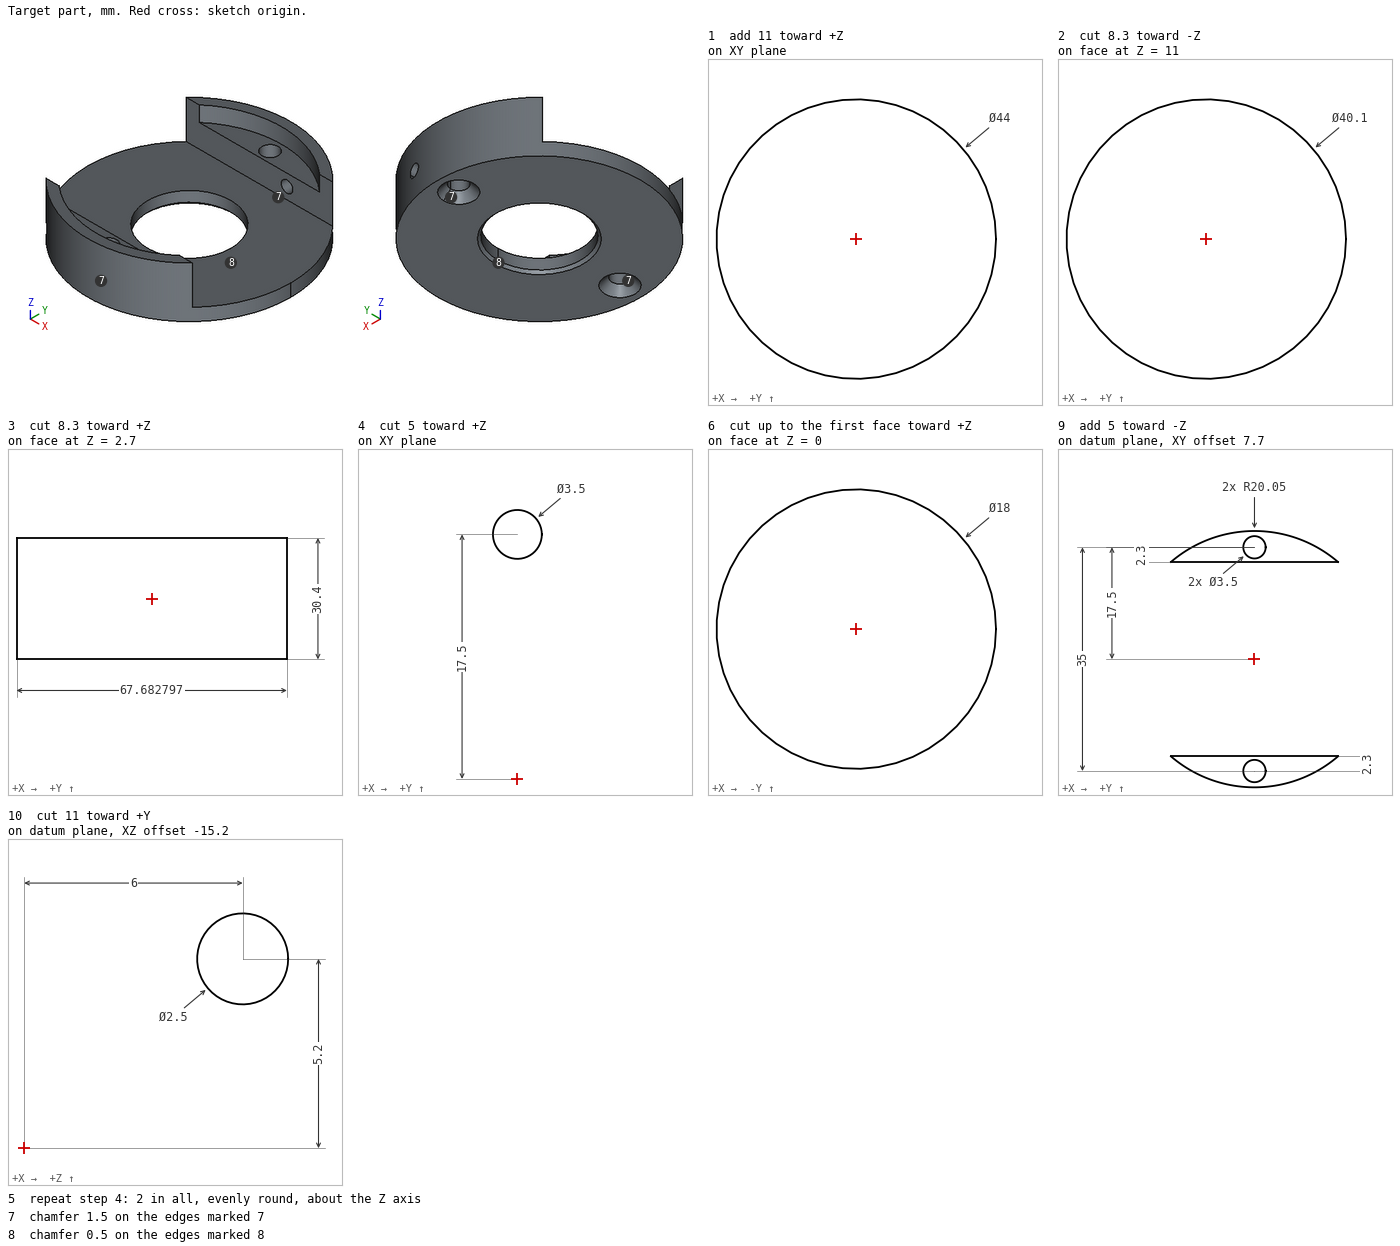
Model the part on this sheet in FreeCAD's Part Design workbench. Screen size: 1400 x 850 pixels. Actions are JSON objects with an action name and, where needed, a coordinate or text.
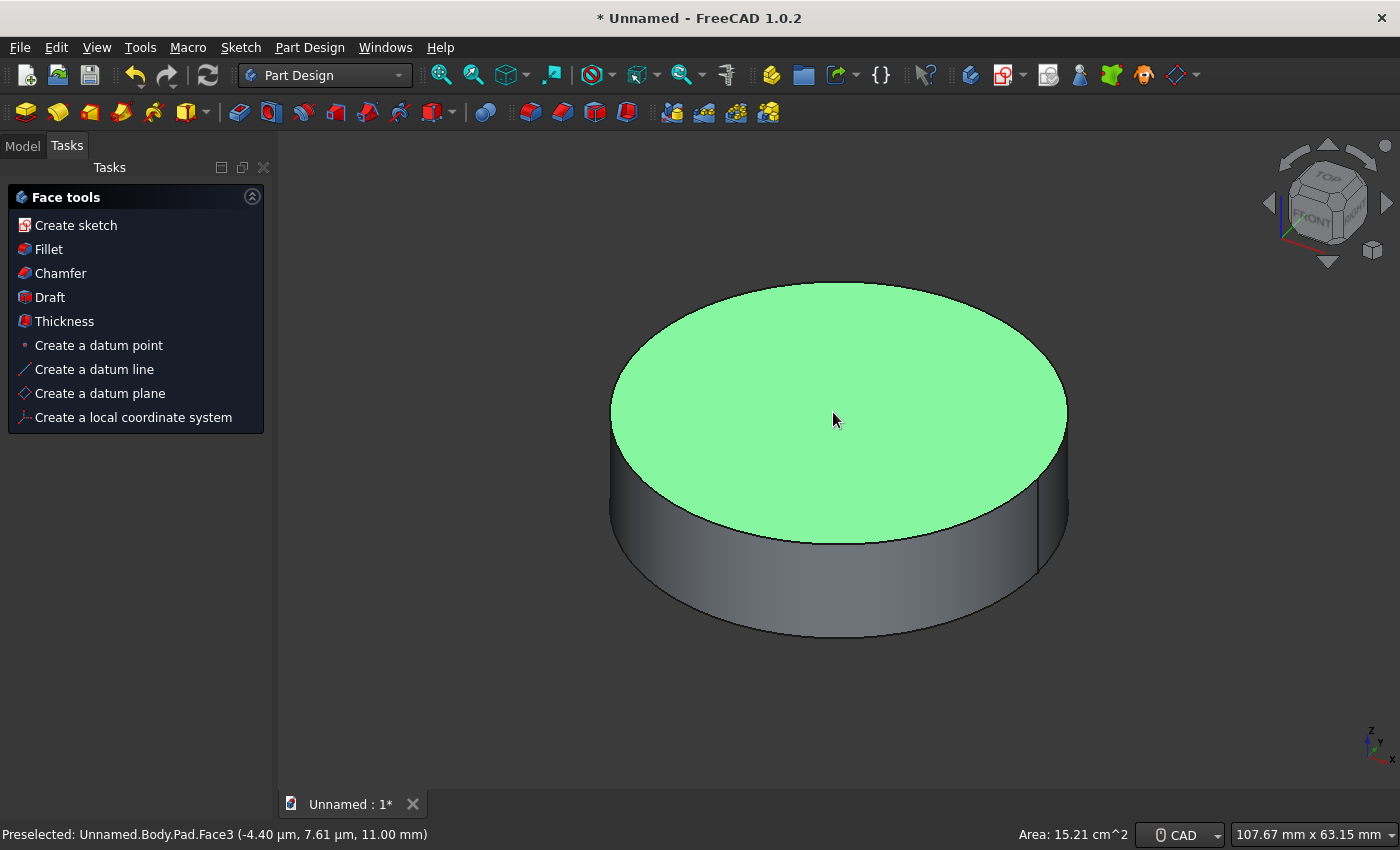
{"action": "left_click", "coordinate": [1004, 76]}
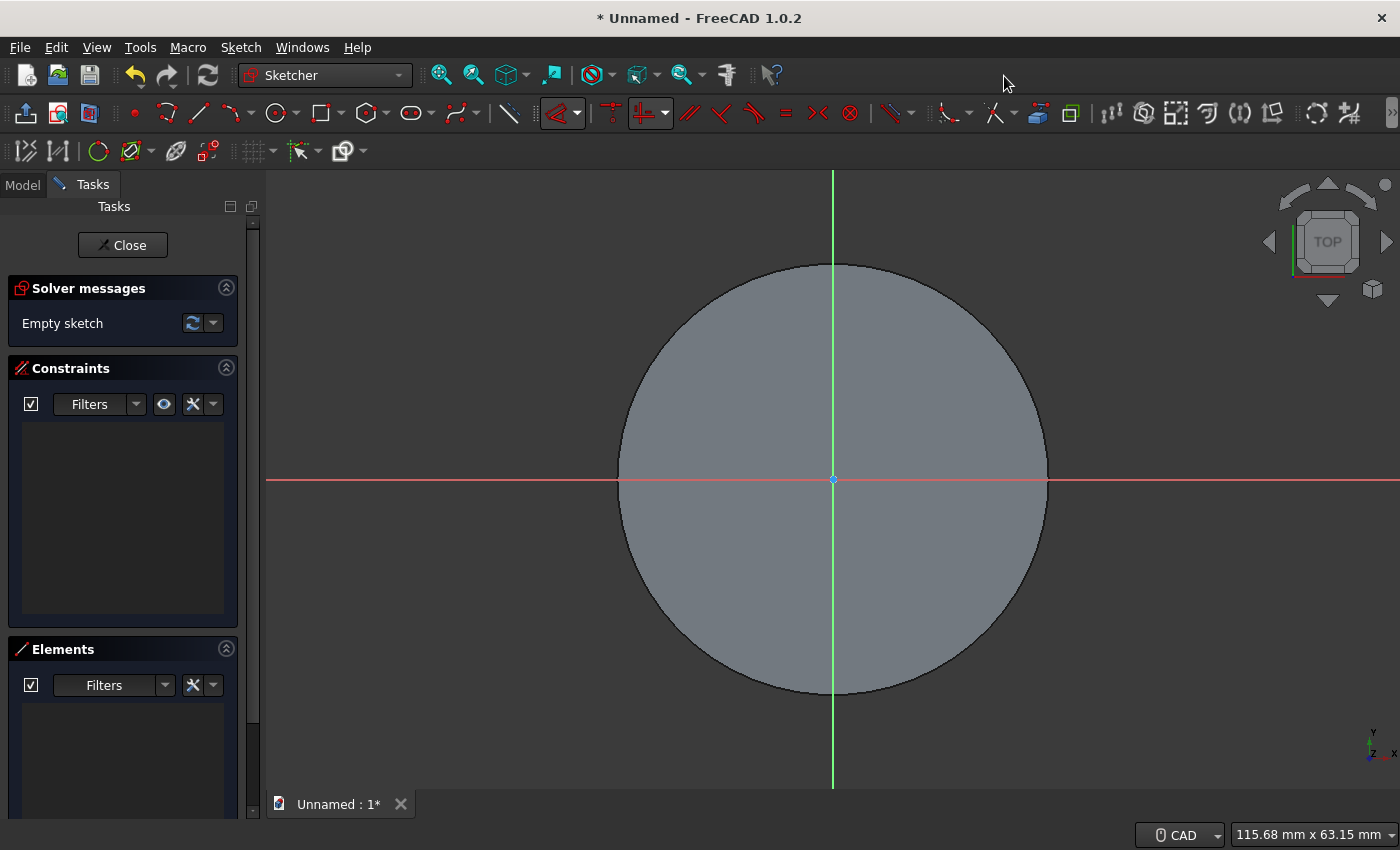
{"action": "key", "text": "g c"}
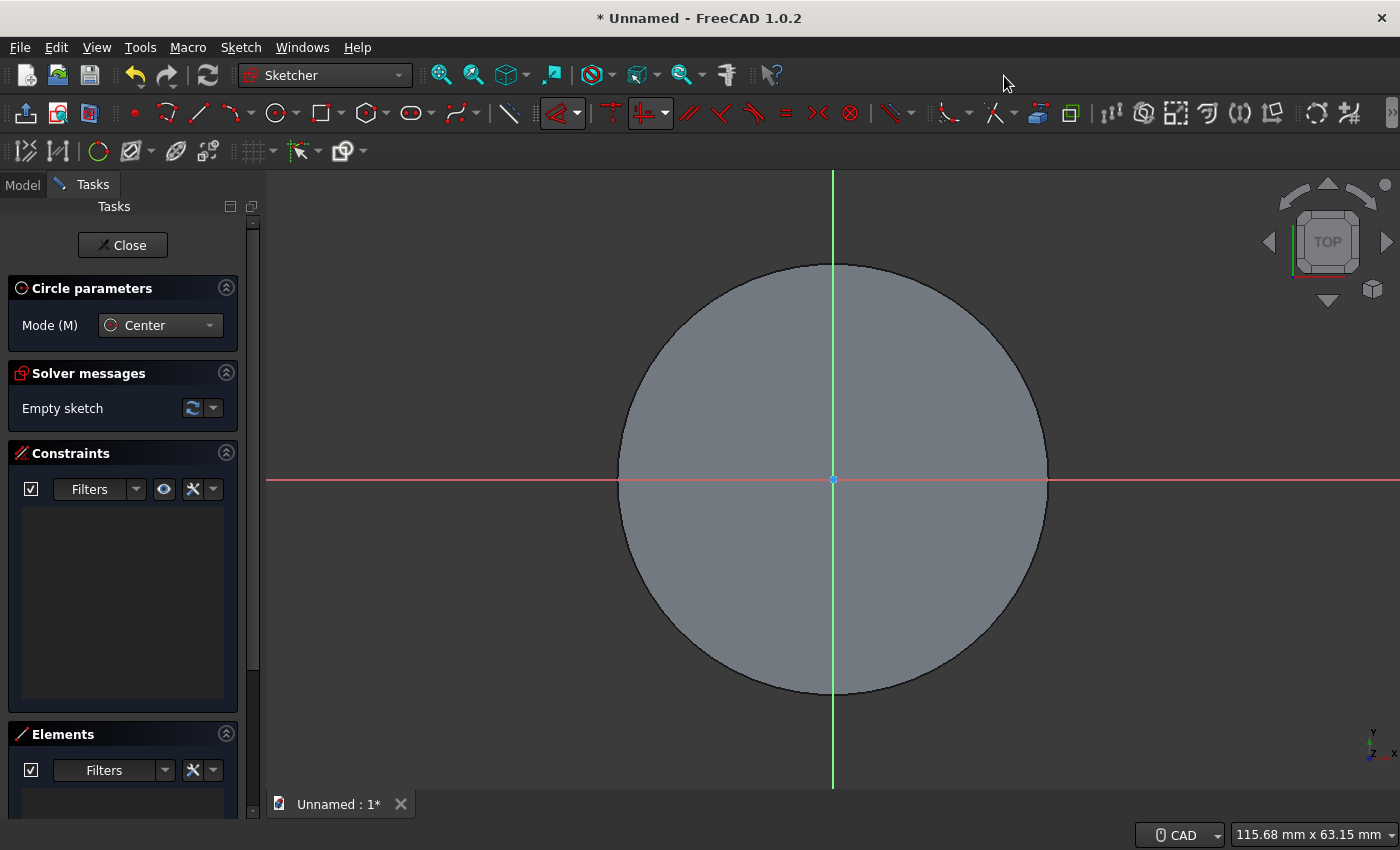
{"action": "left_click", "coordinate": [833, 480]}
{"action": "left_click", "coordinate": [972, 341]}
{"action": "key", "text": "Escape"}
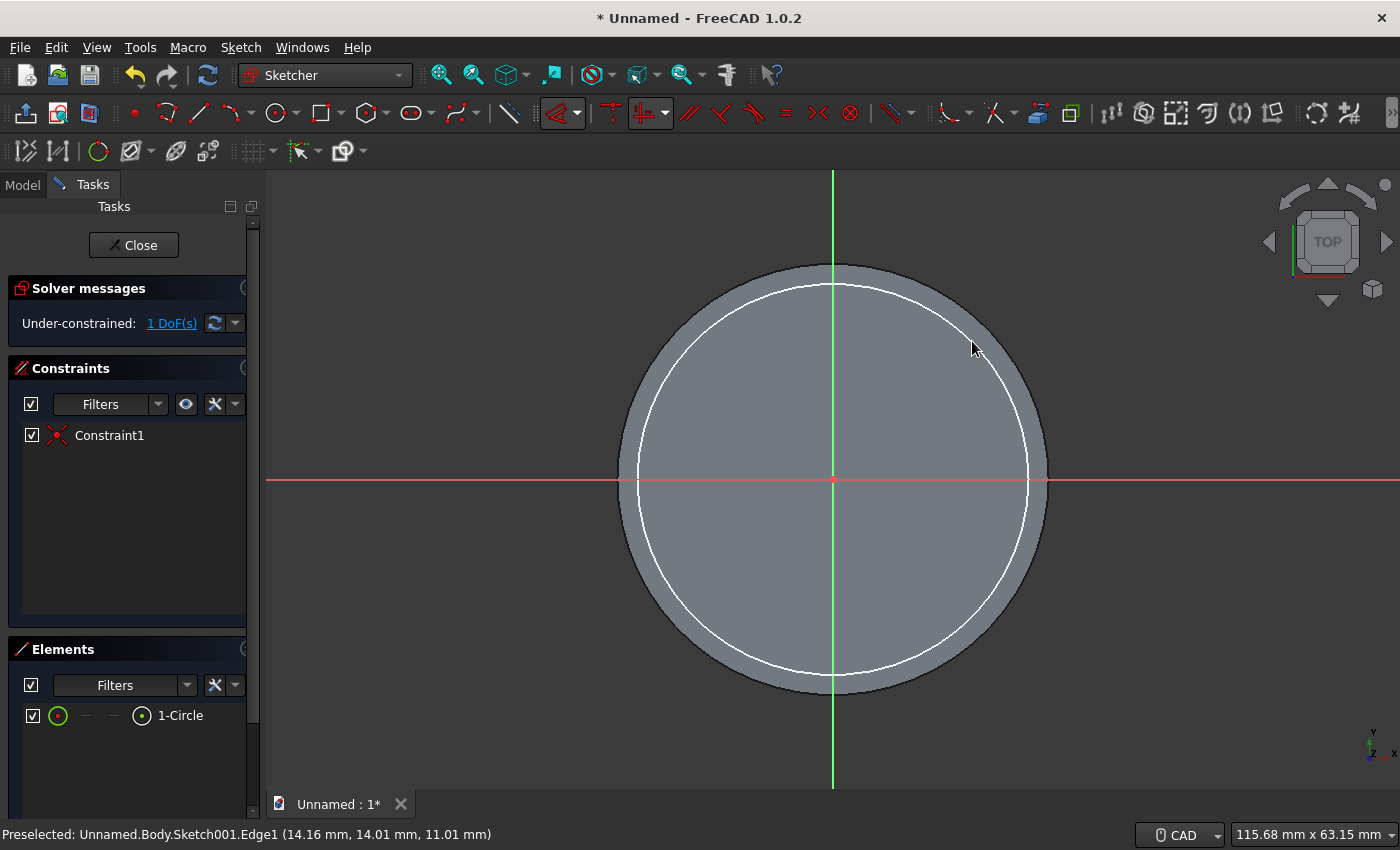
{"action": "left_click", "coordinate": [556, 114]}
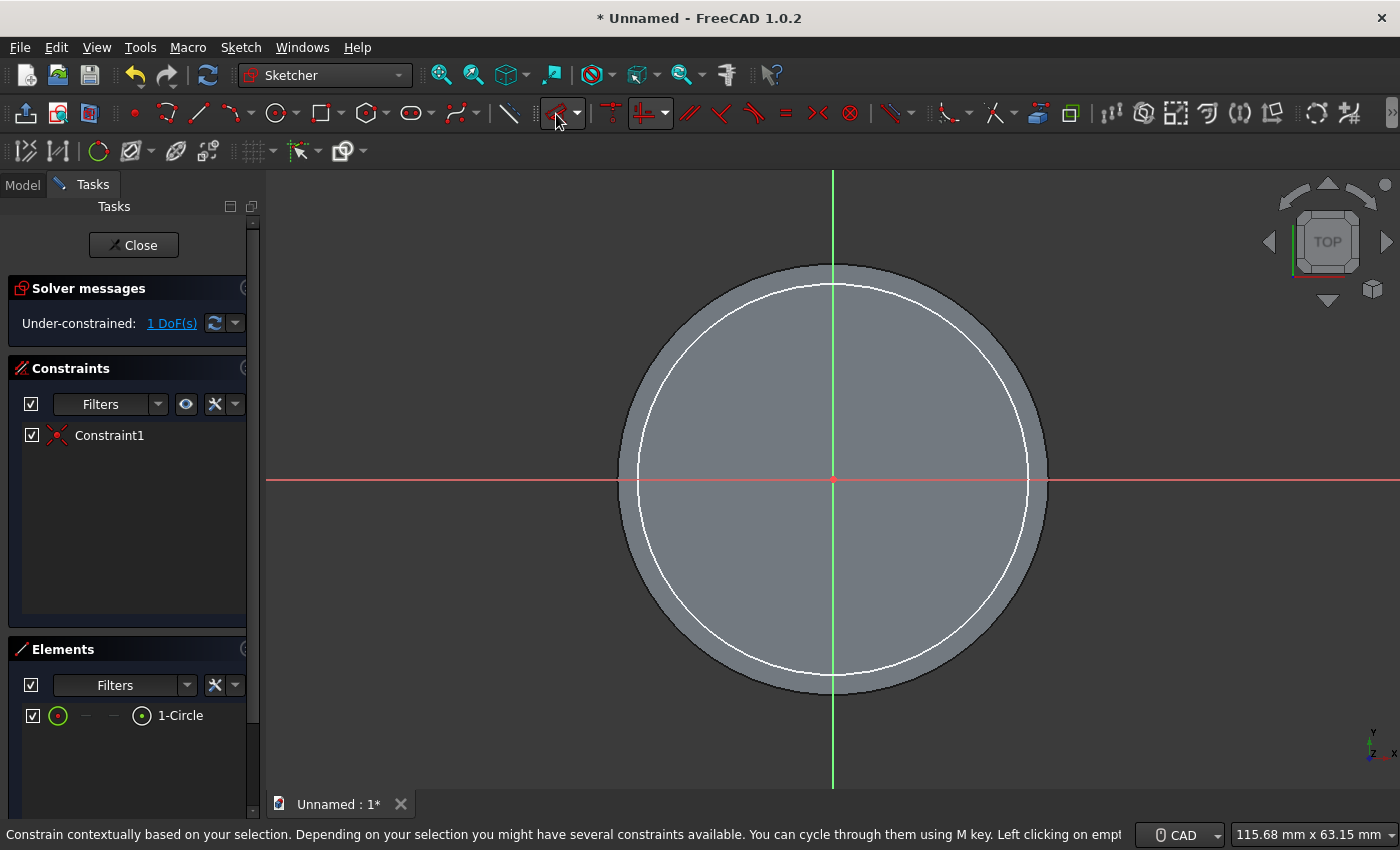
{"action": "left_click", "coordinate": [971, 341]}
{"action": "left_click", "coordinate": [994, 318]}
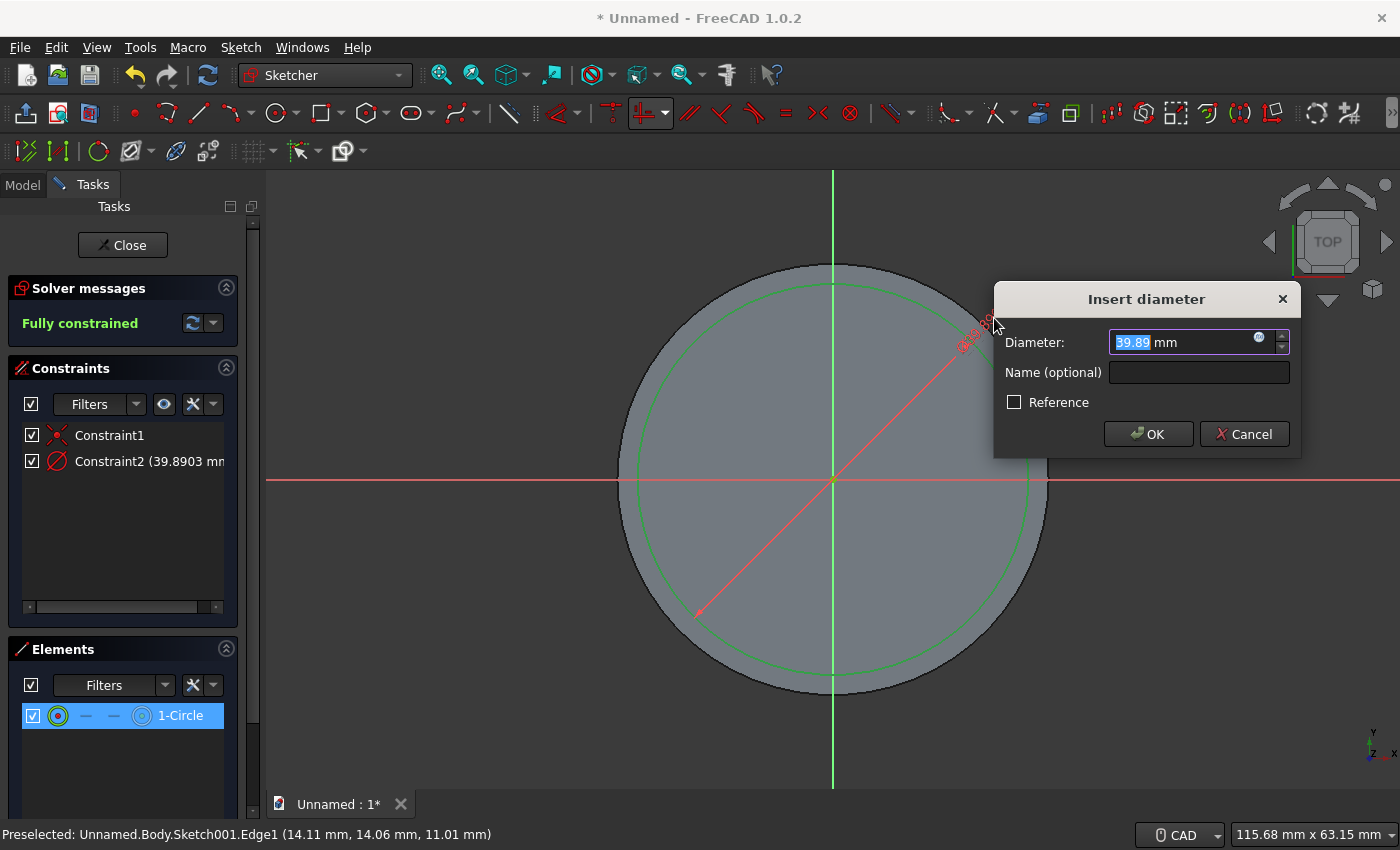
{"action": "type", "text": "40.1"}
{"action": "key", "text": "Return"}
{"action": "key", "text": "Escape"}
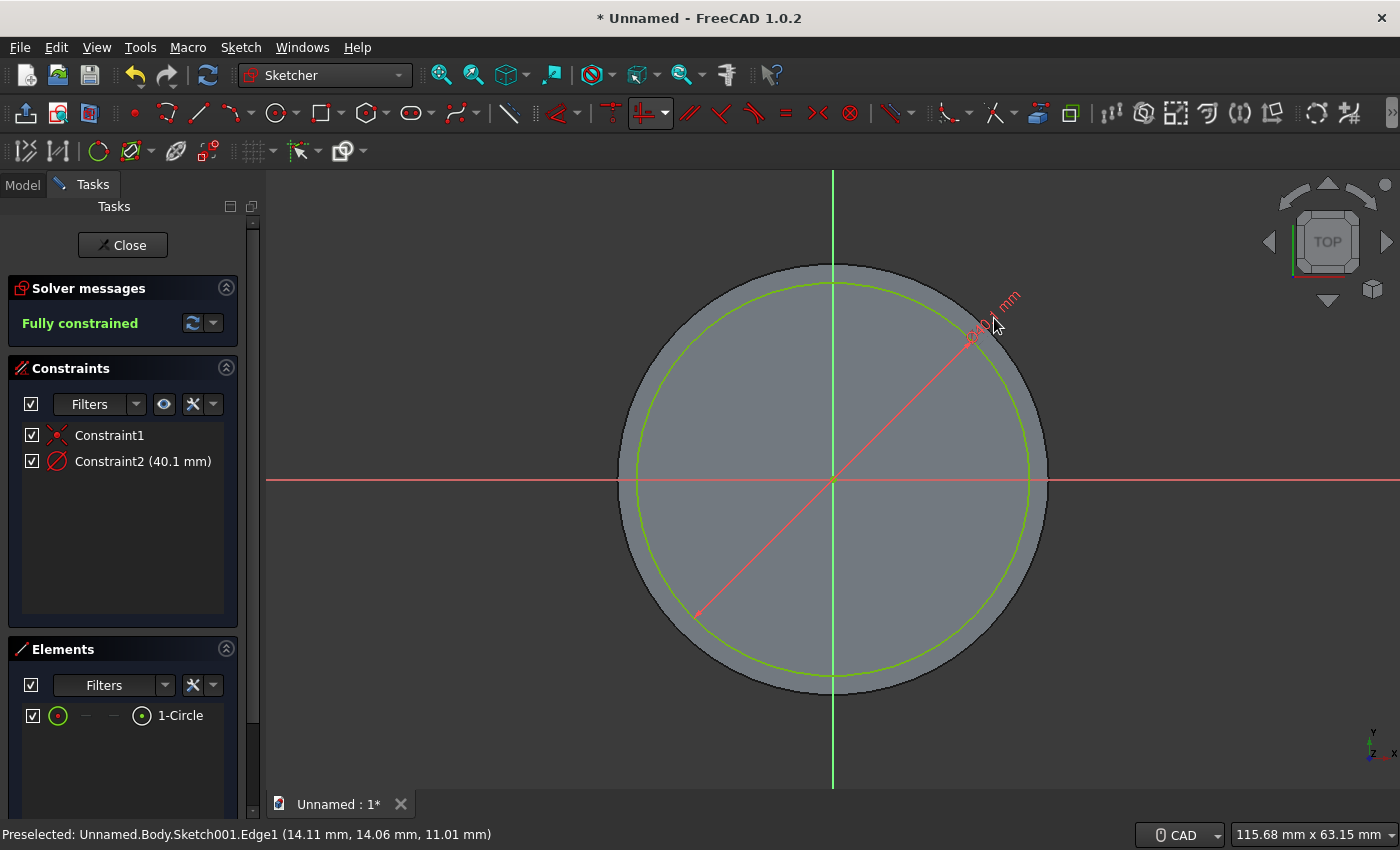
{"action": "left_click", "coordinate": [123, 245]}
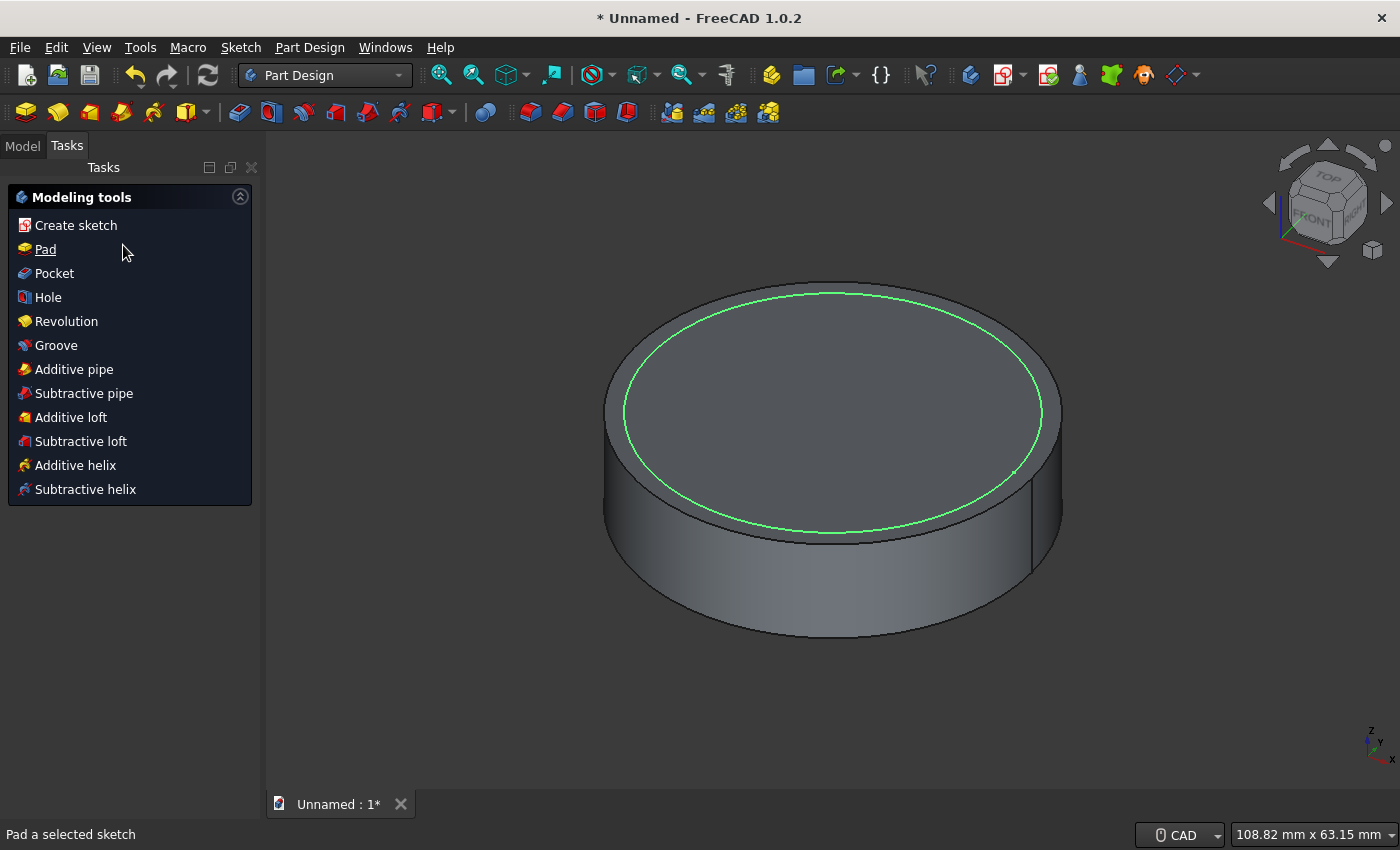
{"action": "left_click", "coordinate": [240, 112]}